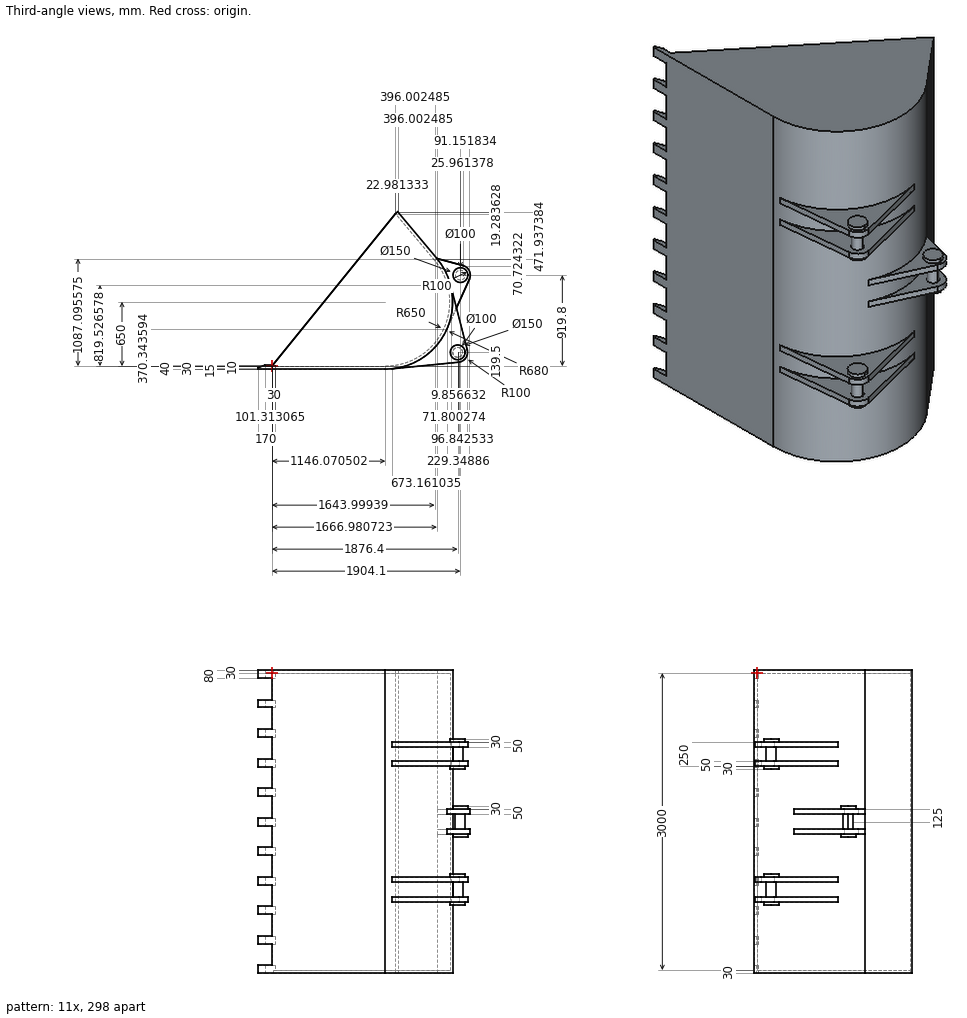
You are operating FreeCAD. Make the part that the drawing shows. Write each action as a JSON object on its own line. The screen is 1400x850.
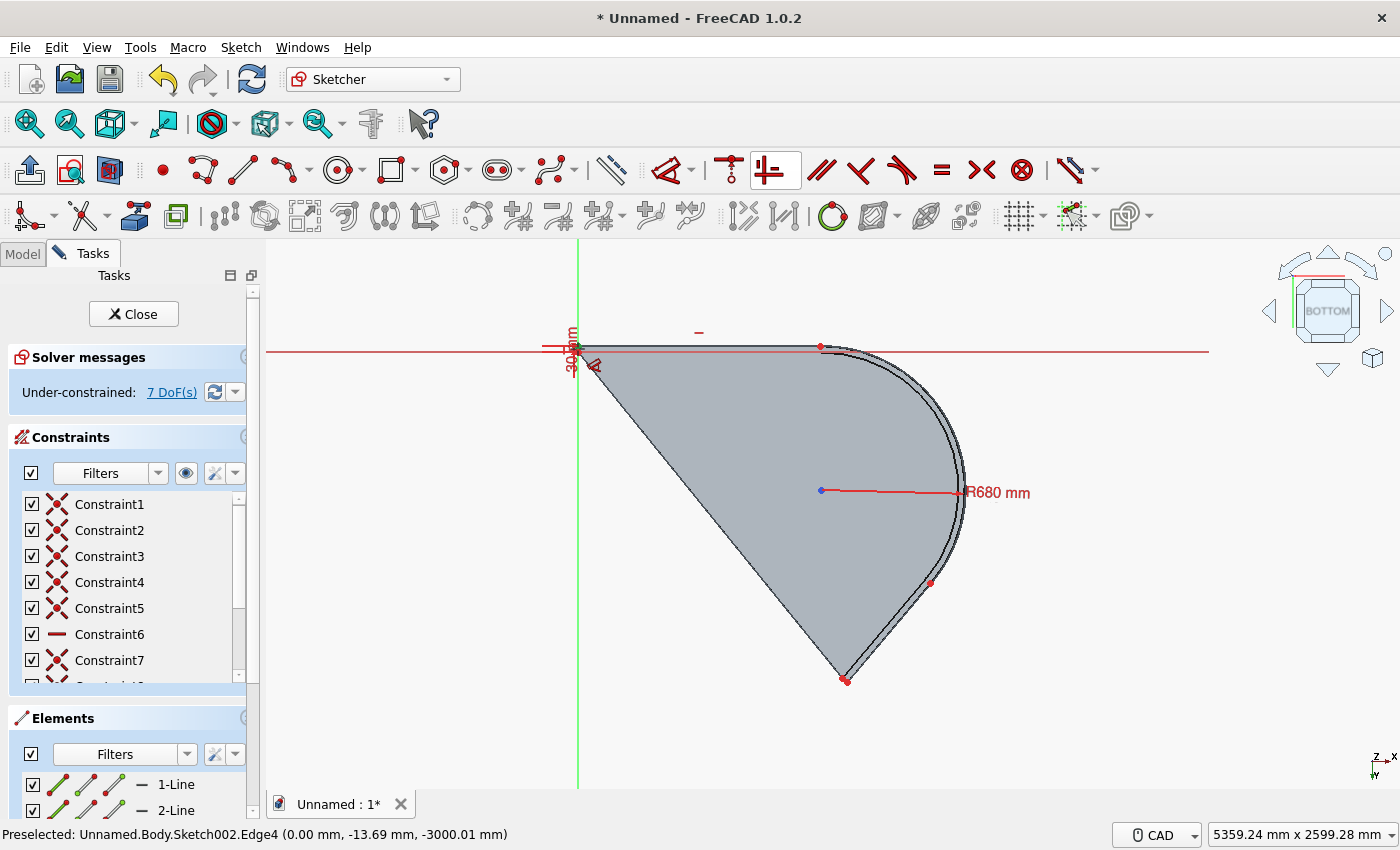
{"action": "scroll", "coordinate": [846, 682], "scroll_direction": "up", "scroll_amount": 11}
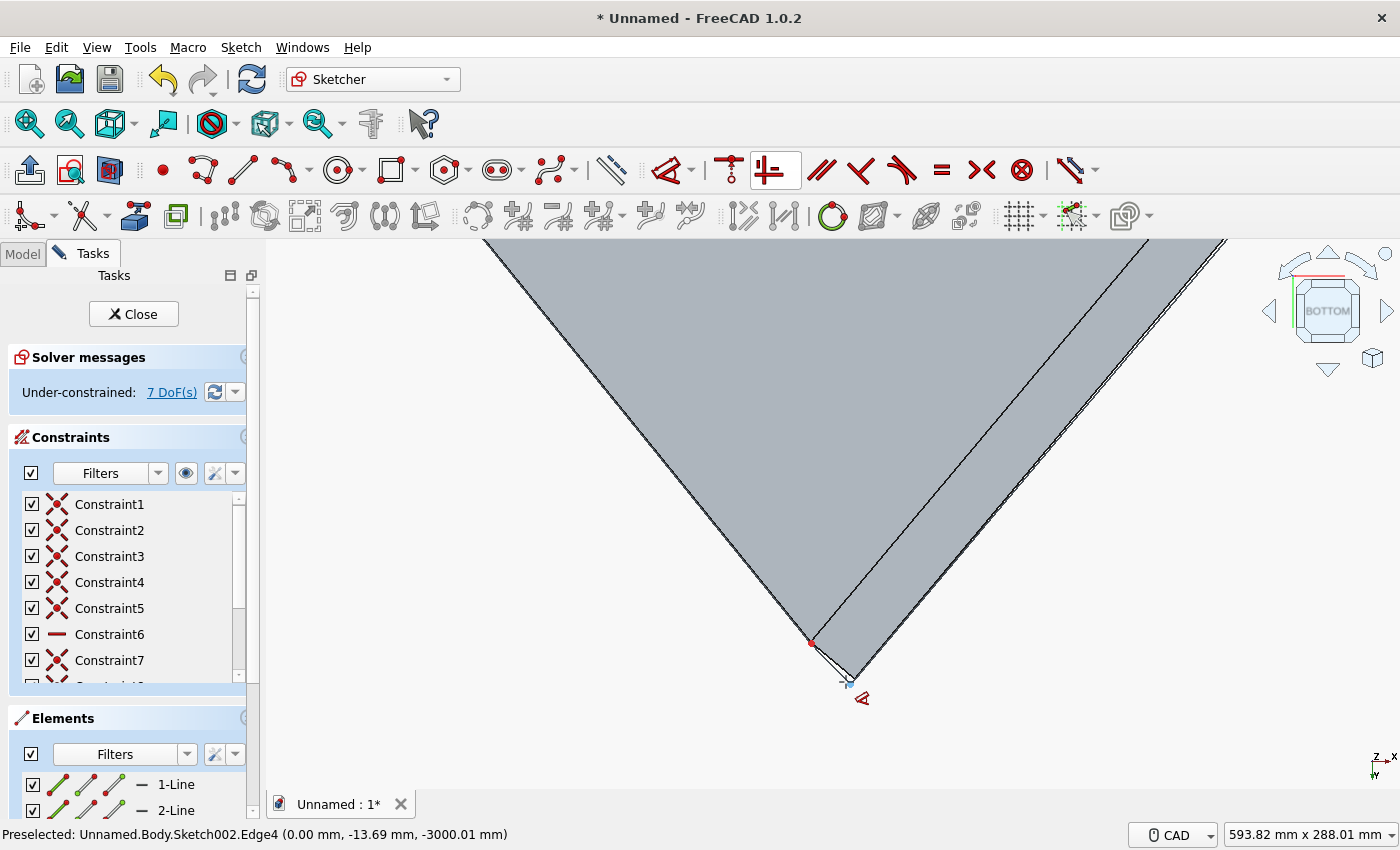
{"action": "left_click", "coordinate": [839, 672]}
{"action": "left_click", "coordinate": [831, 719]}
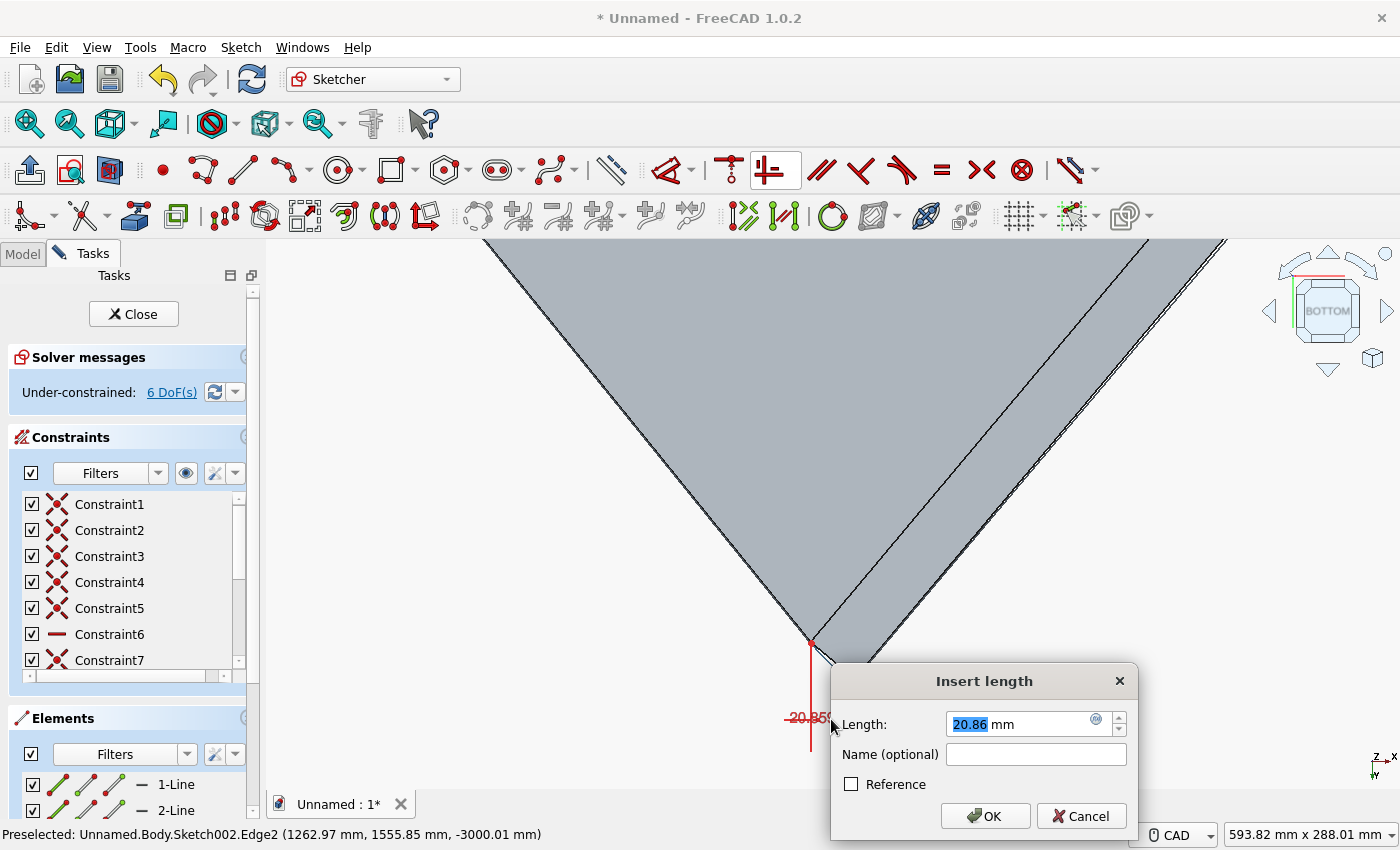
{"action": "type", "text": "22.981333"}
{"action": "key", "text": "Return"}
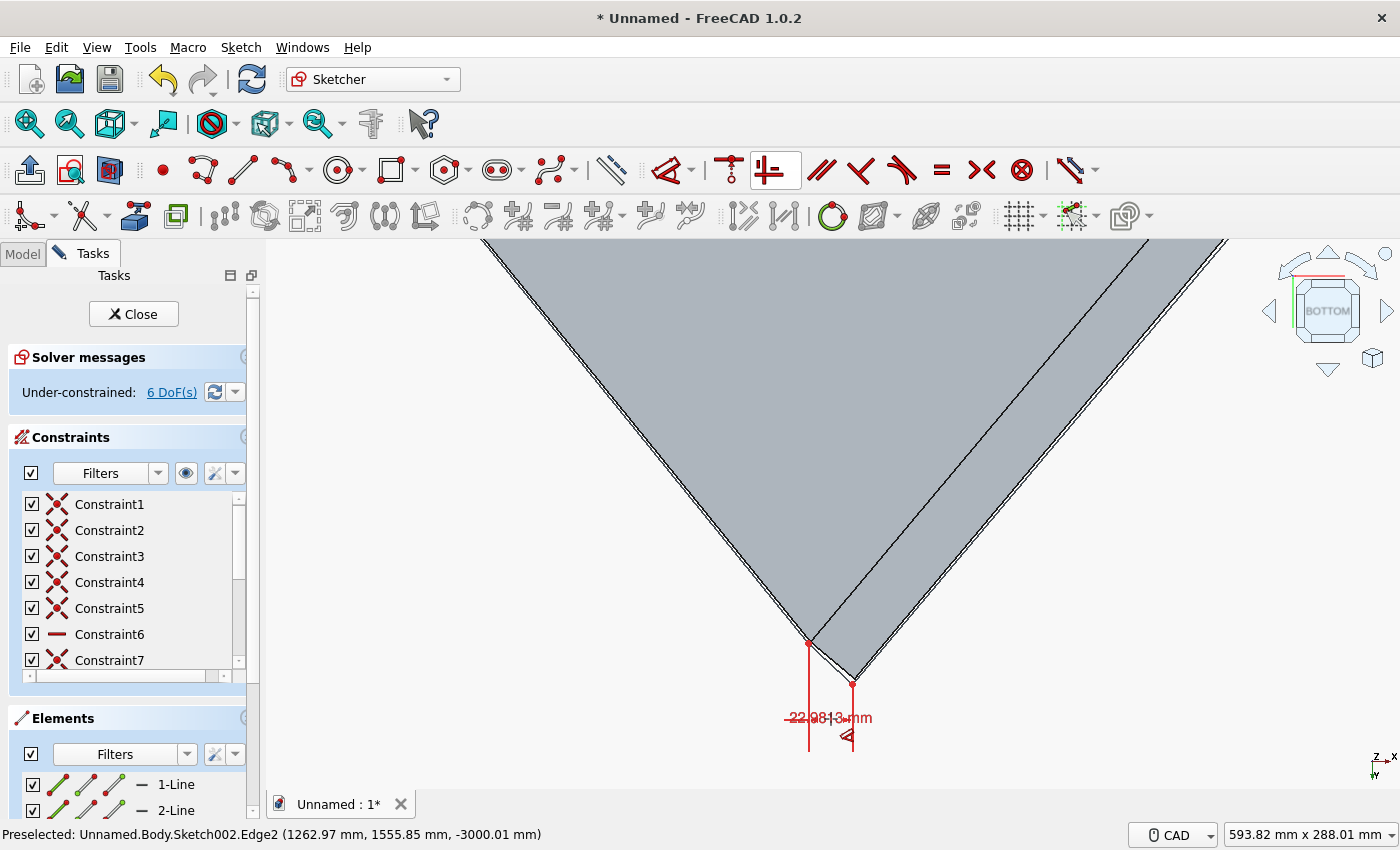
{"action": "left_click", "coordinate": [840, 672]}
{"action": "left_click", "coordinate": [887, 674]}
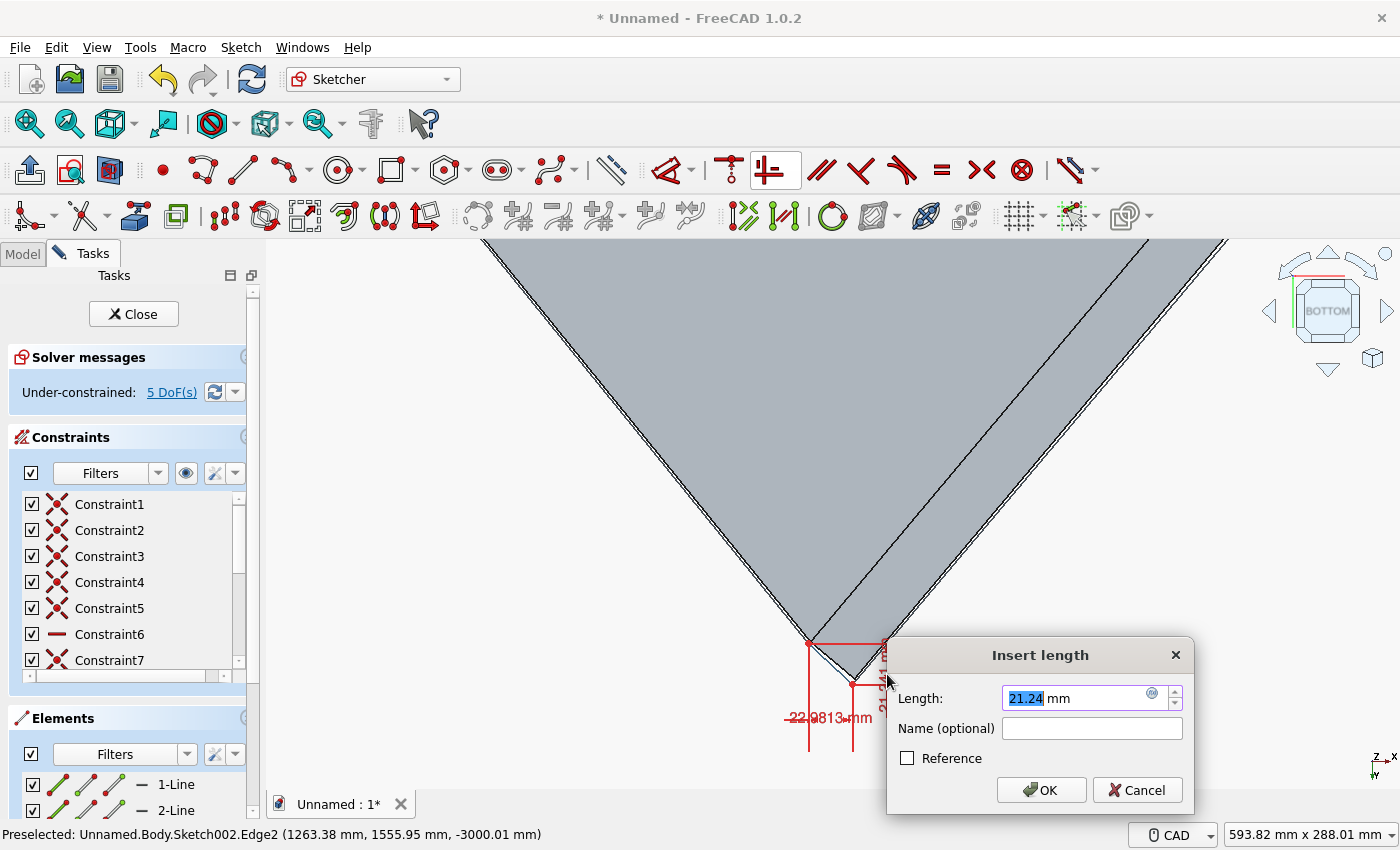
{"action": "type", "text": "19.283628"}
{"action": "key", "text": "Return"}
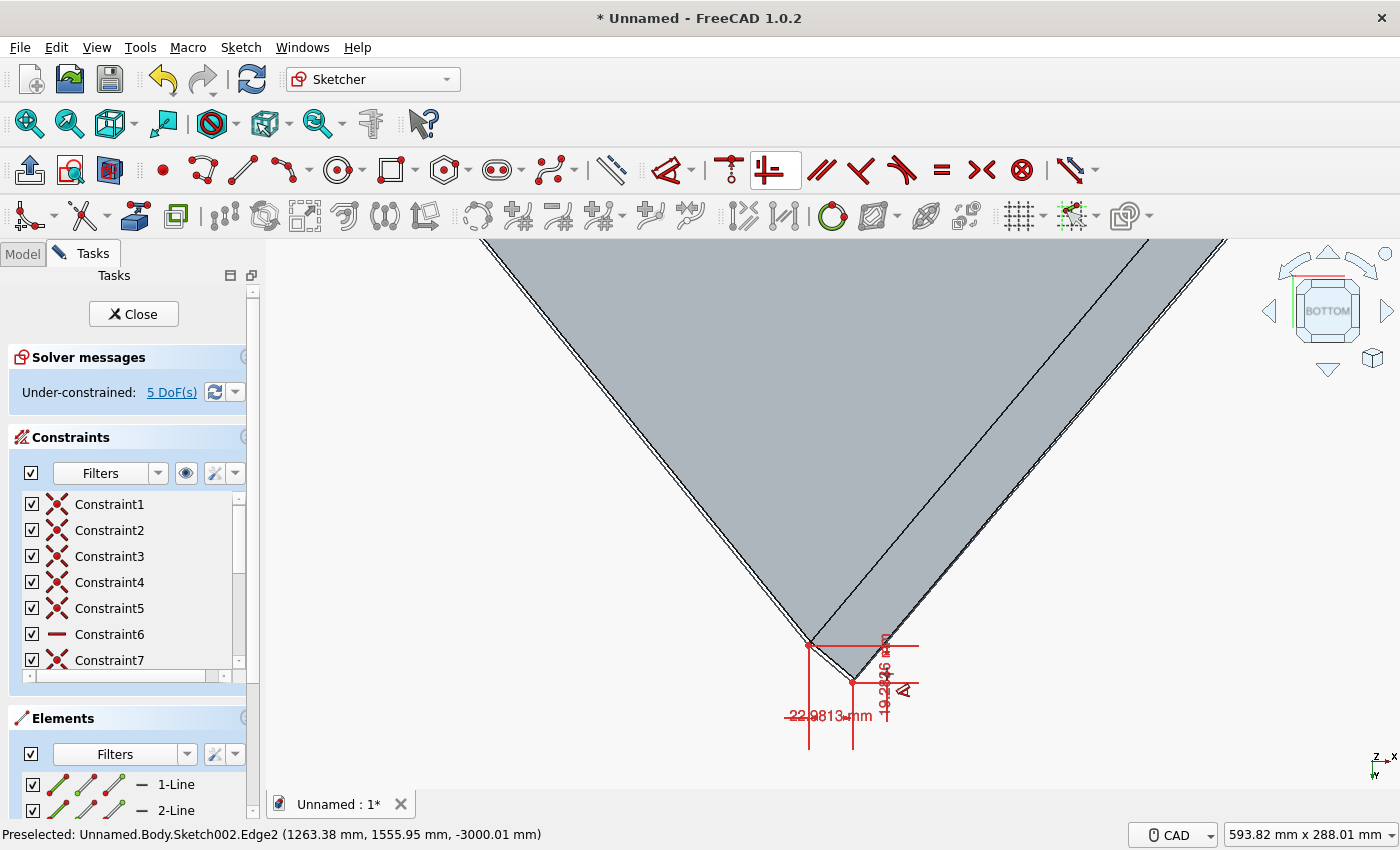
{"action": "scroll", "coordinate": [846, 683], "scroll_direction": "down", "scroll_amount": 11}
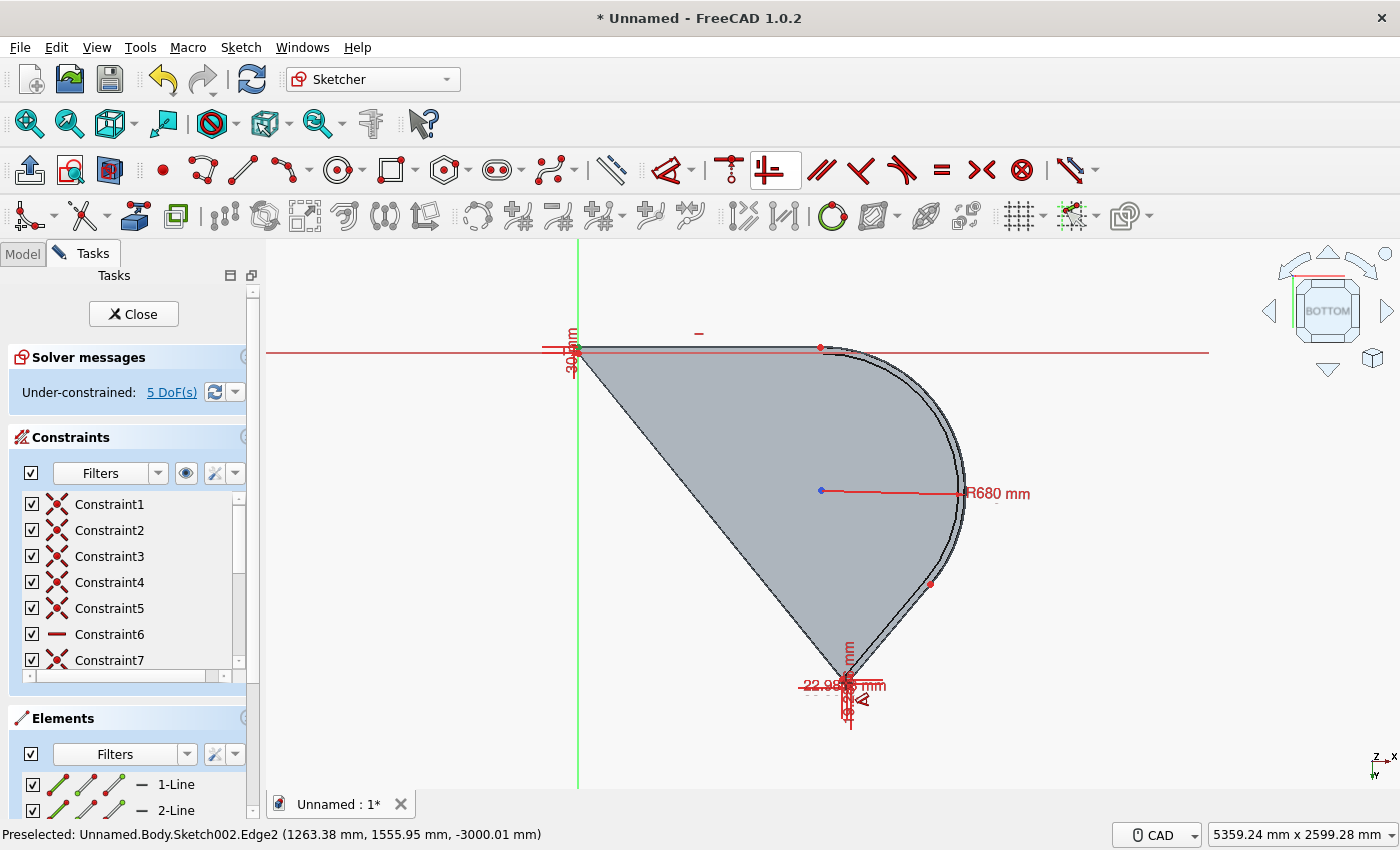
{"action": "scroll", "coordinate": [651, 347], "scroll_direction": "up", "scroll_amount": 4}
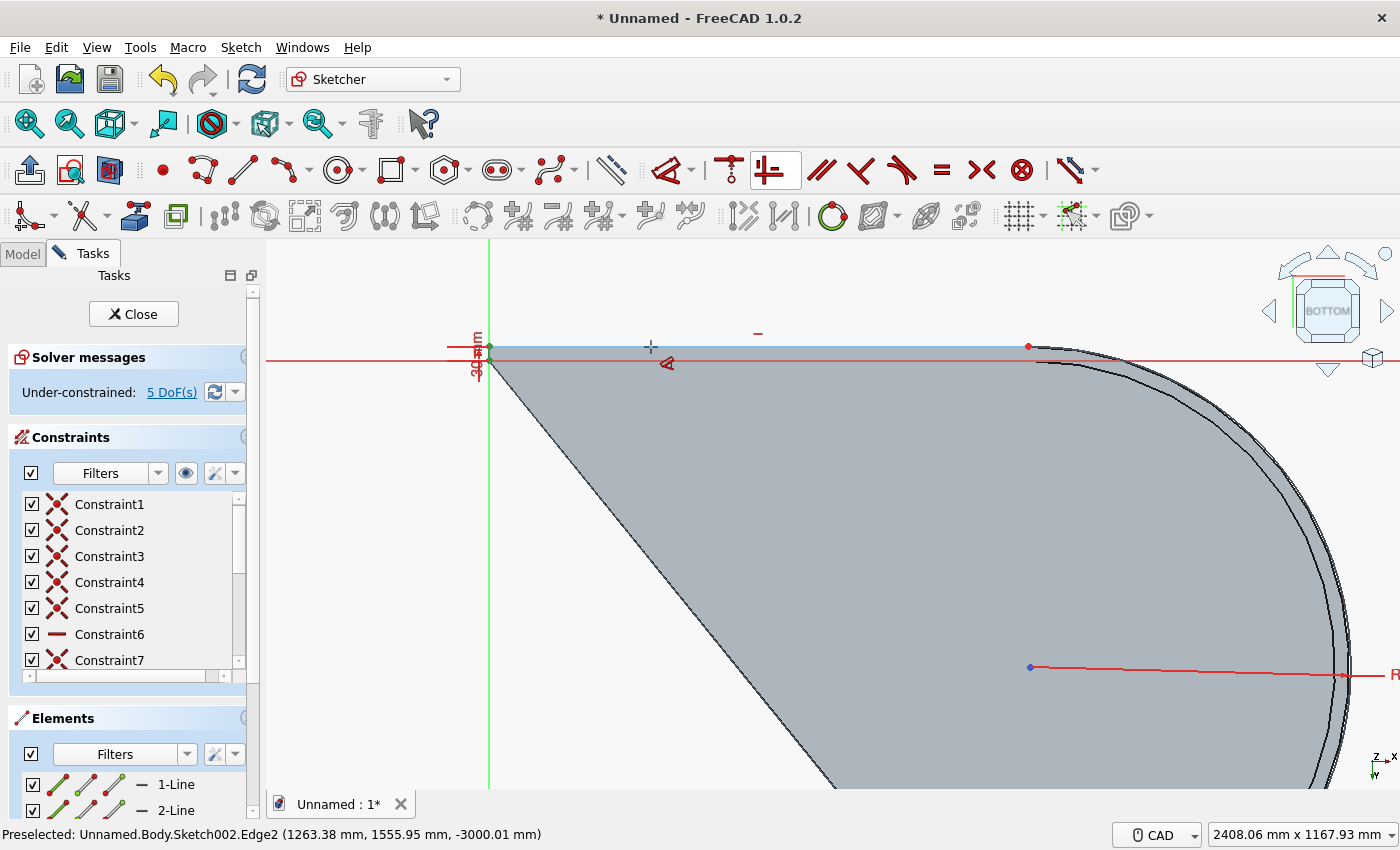
{"action": "left_click", "coordinate": [651, 347]}
{"action": "left_click", "coordinate": [759, 313]}